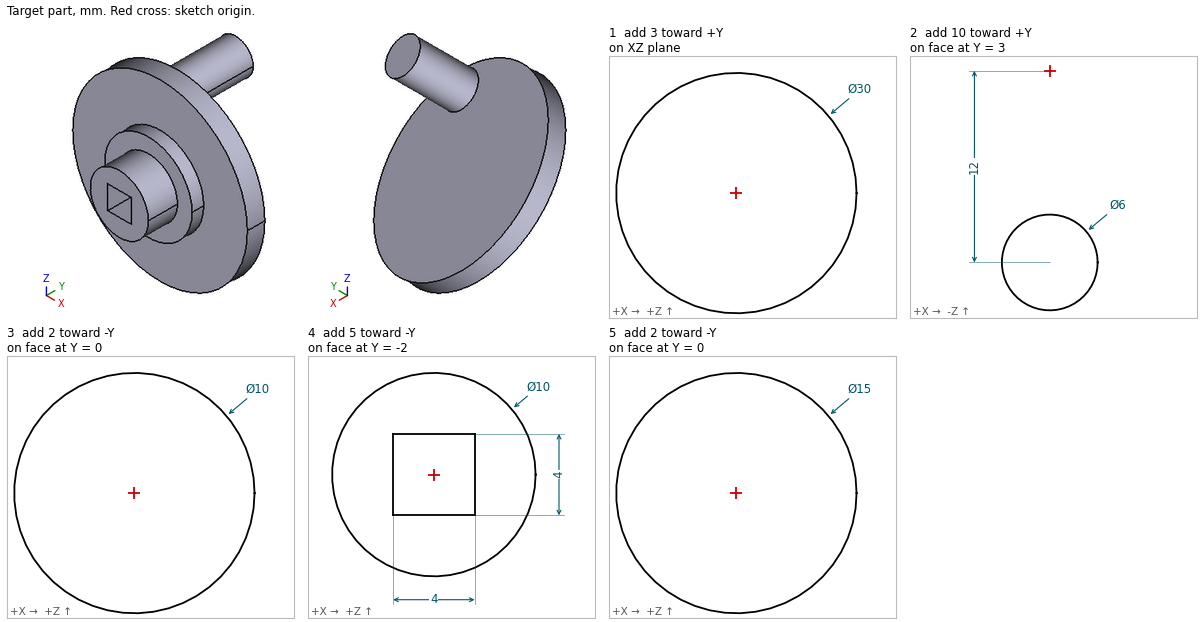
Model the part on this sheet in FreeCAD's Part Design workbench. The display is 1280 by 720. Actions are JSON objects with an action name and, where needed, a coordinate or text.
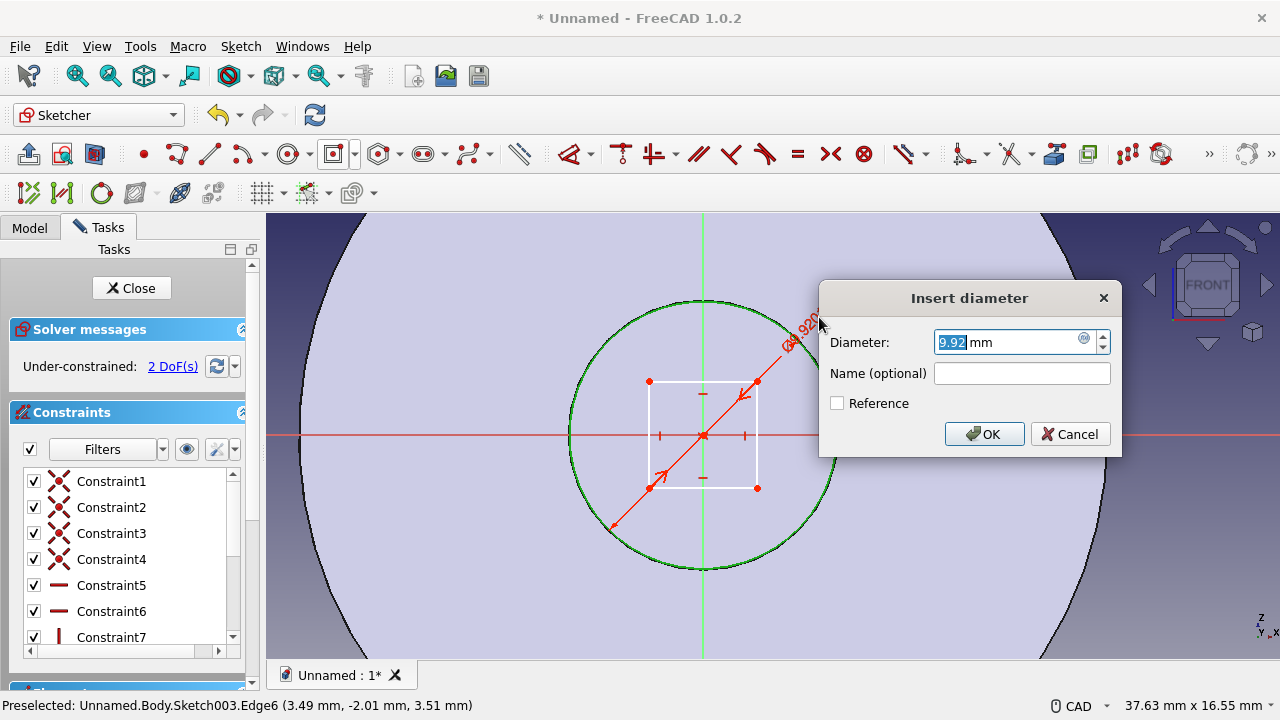
{"action": "type", "text": "10"}
{"action": "key", "text": "Return"}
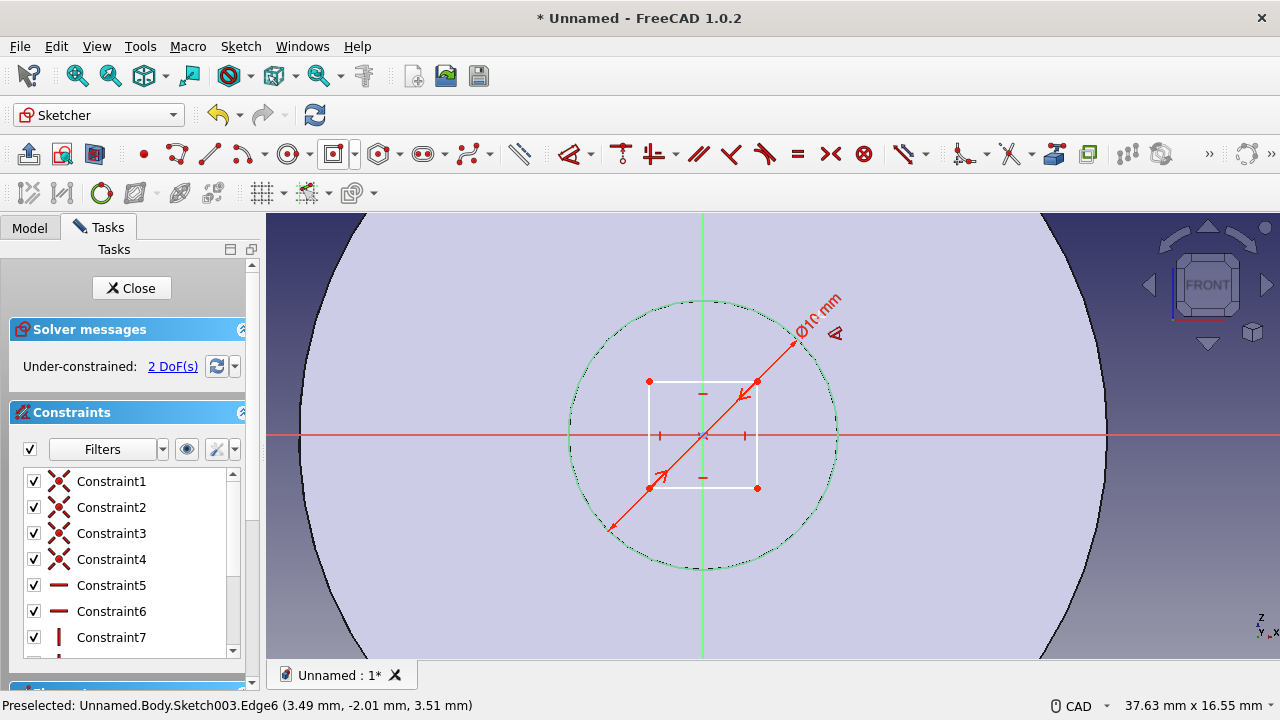
{"action": "left_click", "coordinate": [682, 488]}
{"action": "left_click", "coordinate": [678, 522]}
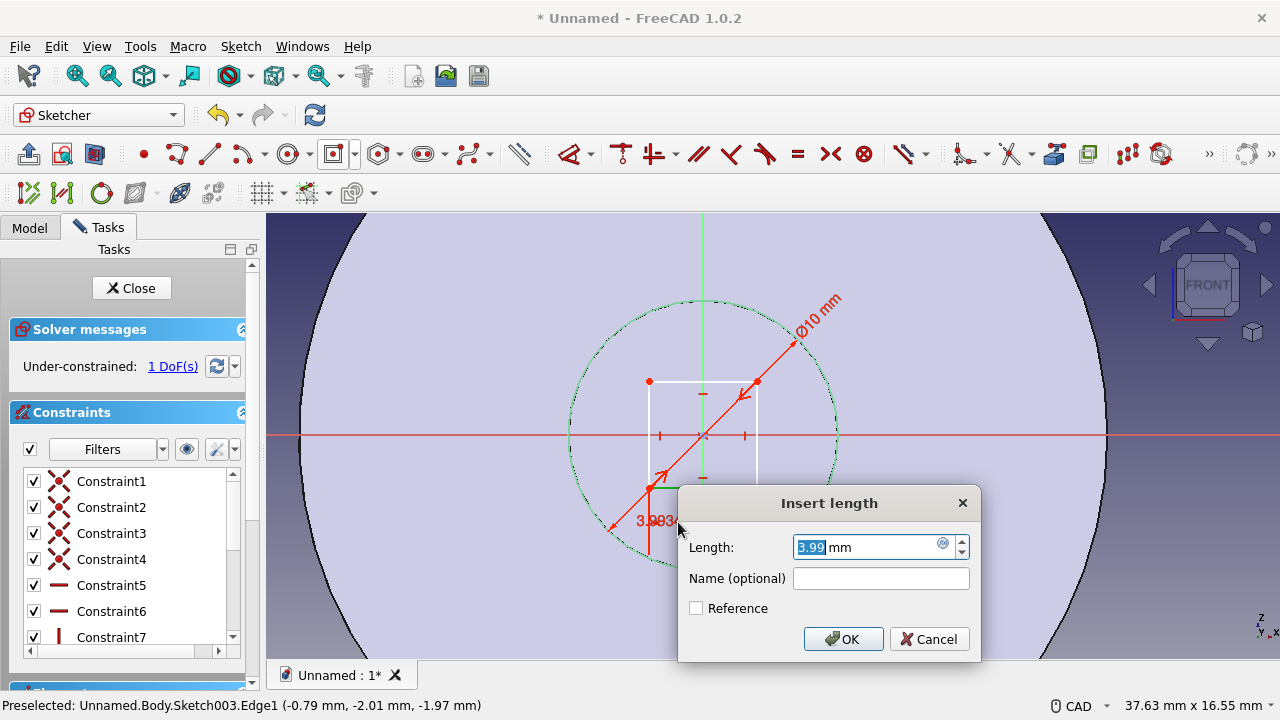
{"action": "type", "text": "4"}
{"action": "key", "text": "Return"}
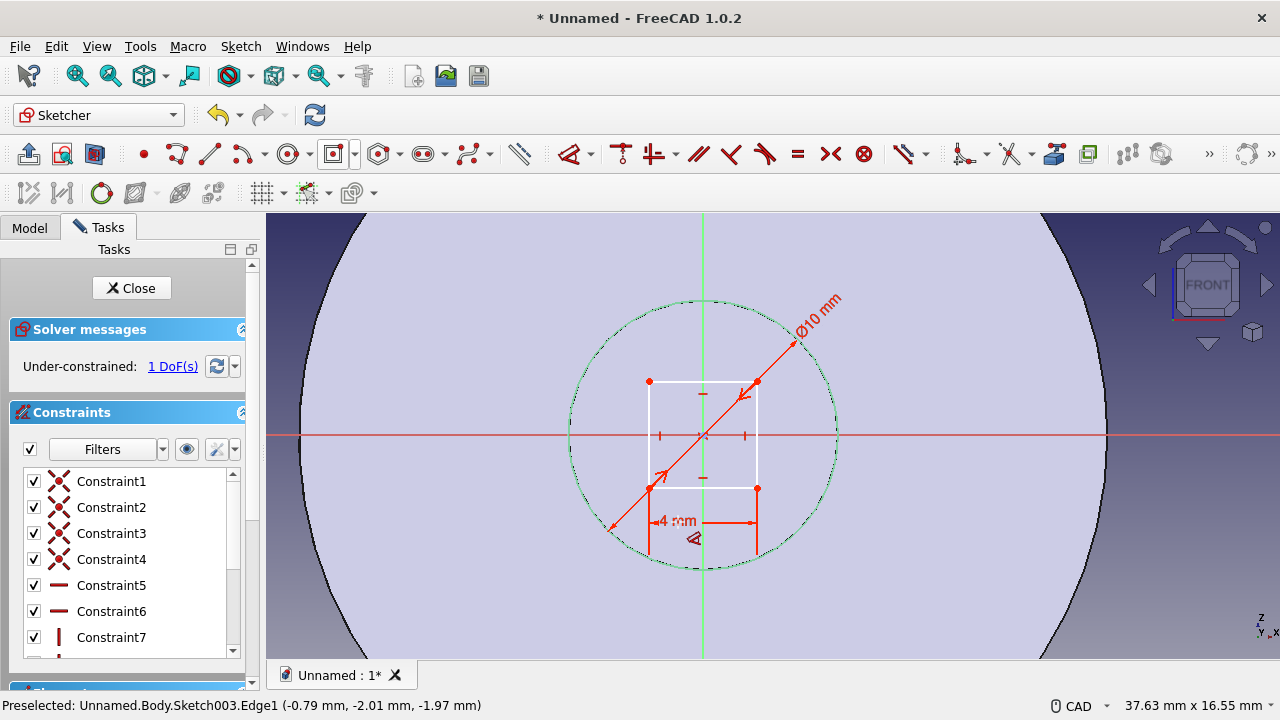
{"action": "left_click", "coordinate": [757, 457]}
{"action": "left_click", "coordinate": [791, 411]}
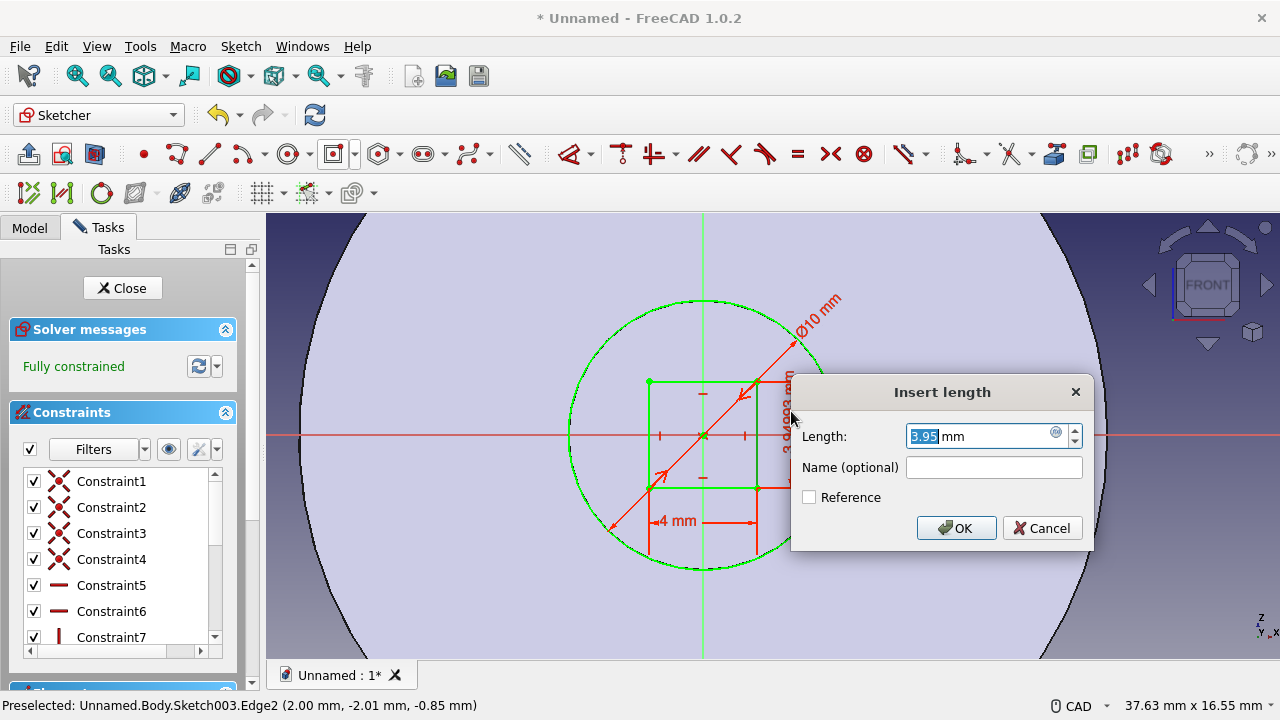
{"action": "type", "text": "4"}
{"action": "key", "text": "Return"}
{"action": "key", "text": "Escape"}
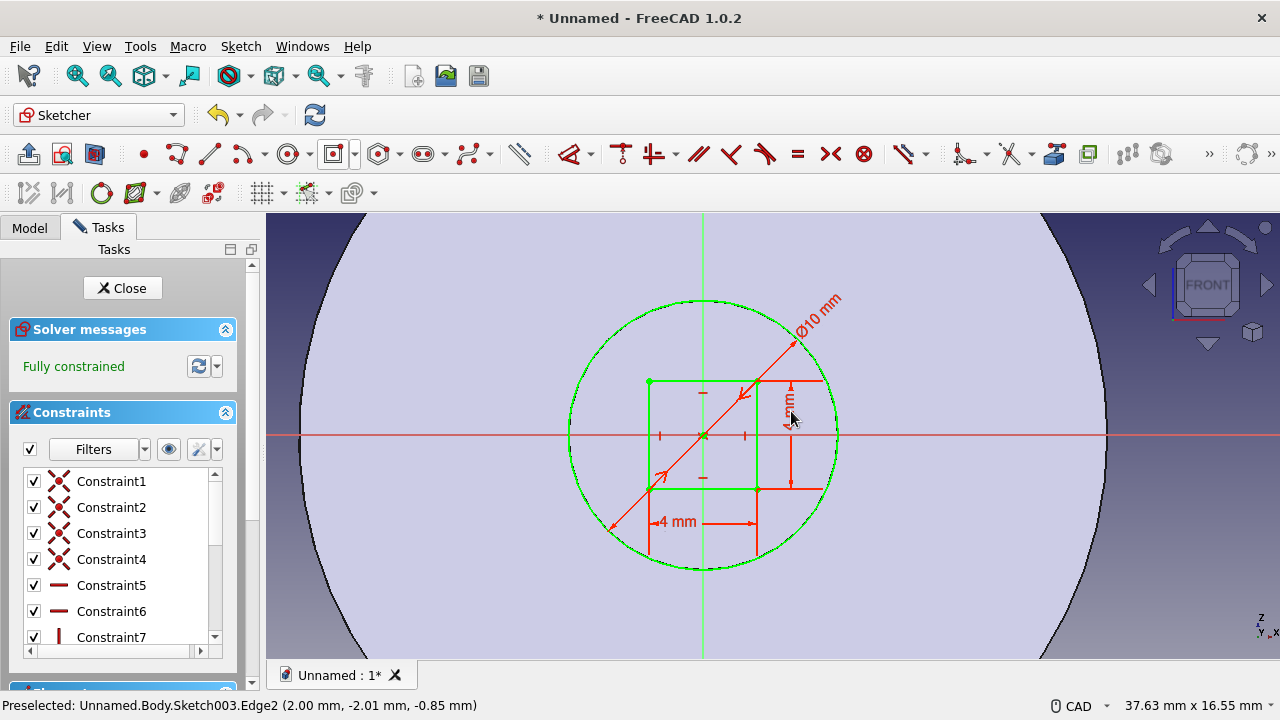
{"action": "left_click", "coordinate": [123, 288]}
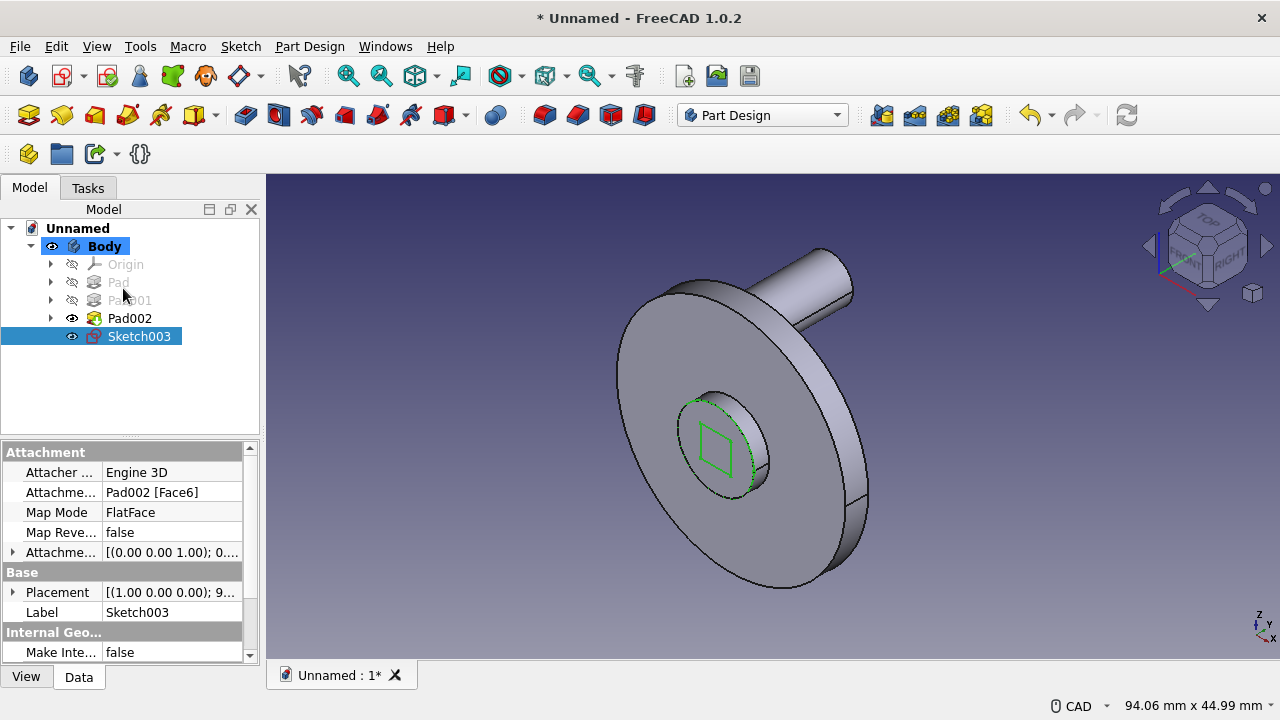
{"action": "left_click", "coordinate": [29, 116]}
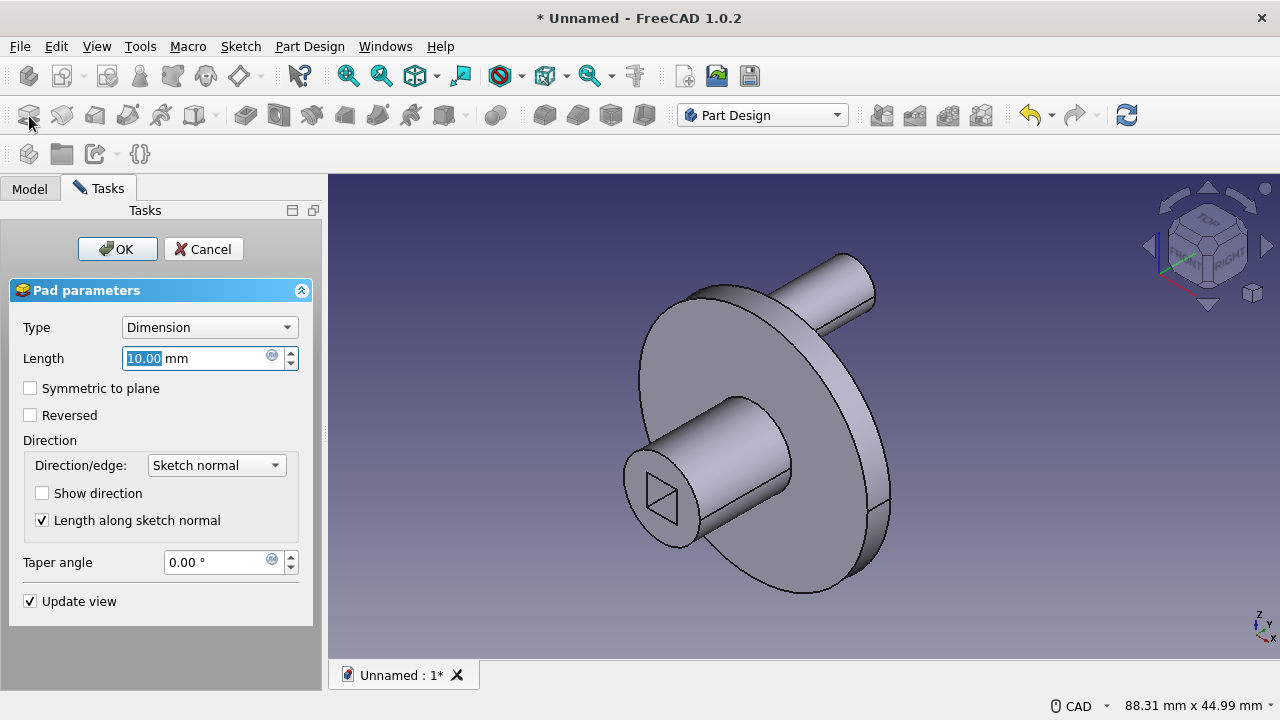
{"action": "type", "text": "5"}
{"action": "key", "text": "Tab"}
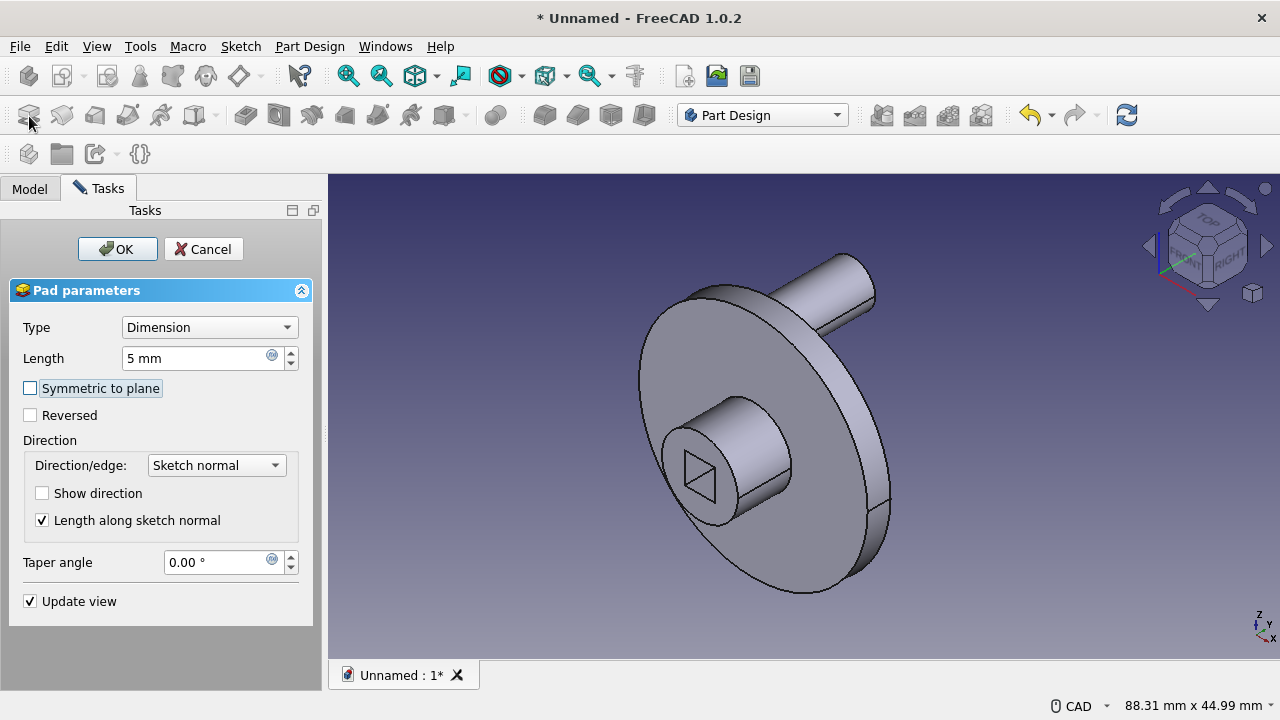
{"action": "left_click", "coordinate": [118, 249]}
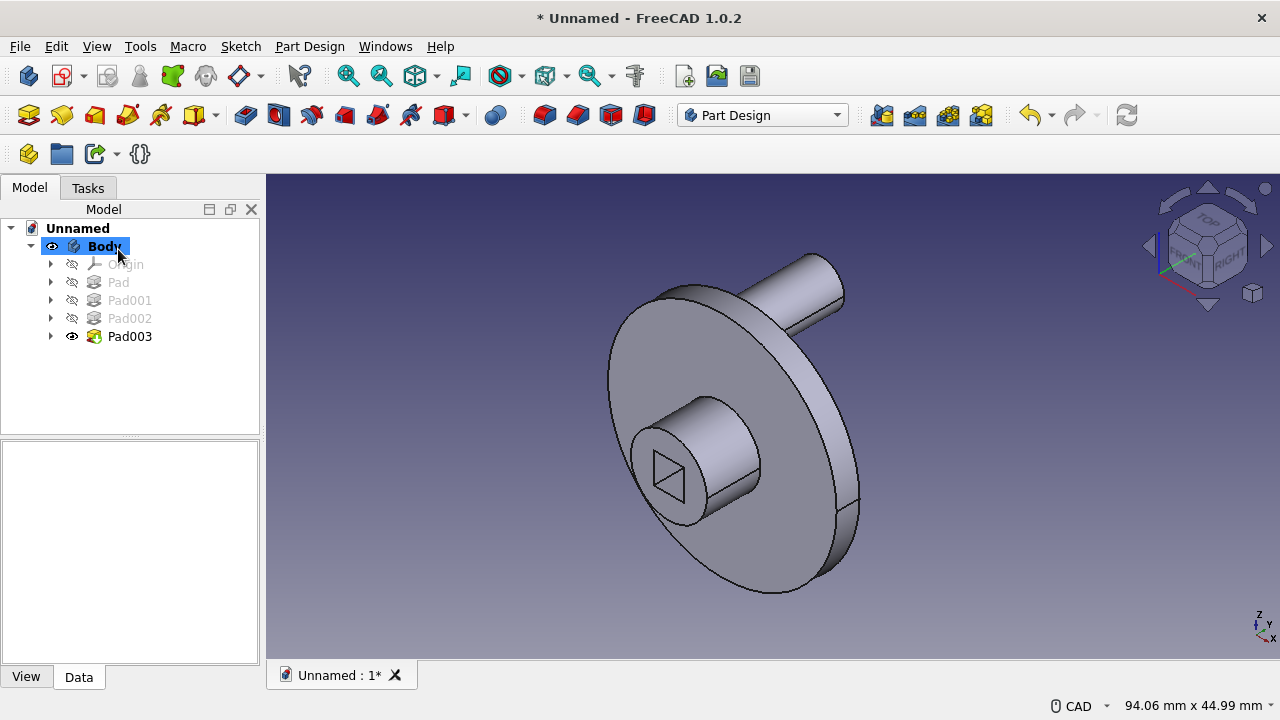
{"action": "left_click", "coordinate": [349, 76]}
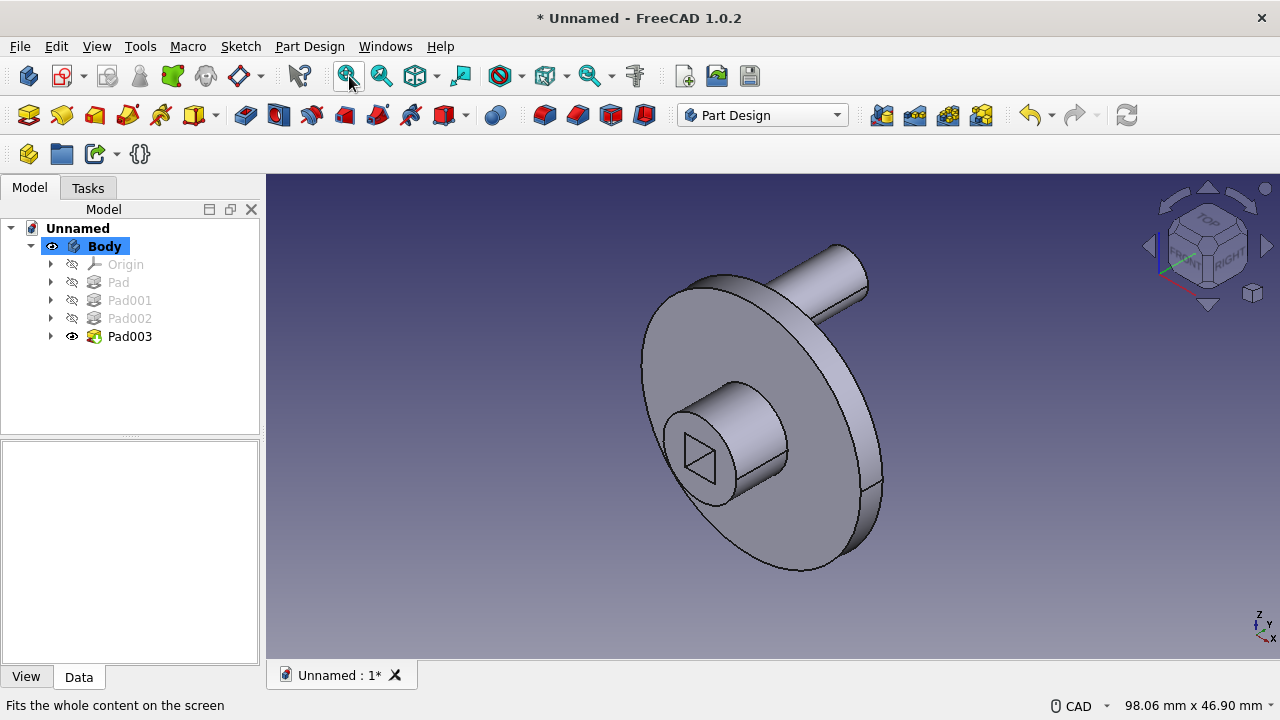
{"action": "left_click", "coordinate": [720, 338]}